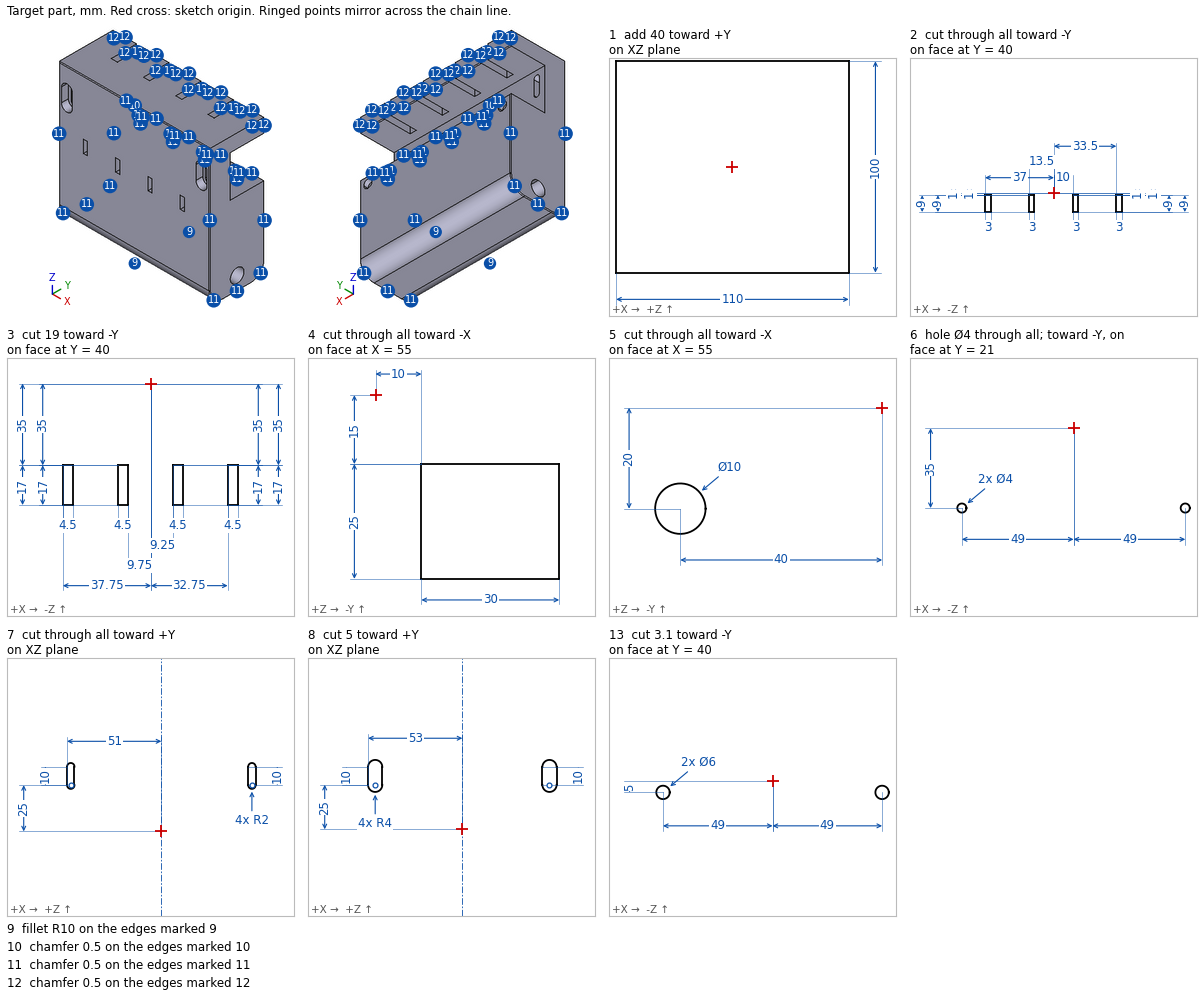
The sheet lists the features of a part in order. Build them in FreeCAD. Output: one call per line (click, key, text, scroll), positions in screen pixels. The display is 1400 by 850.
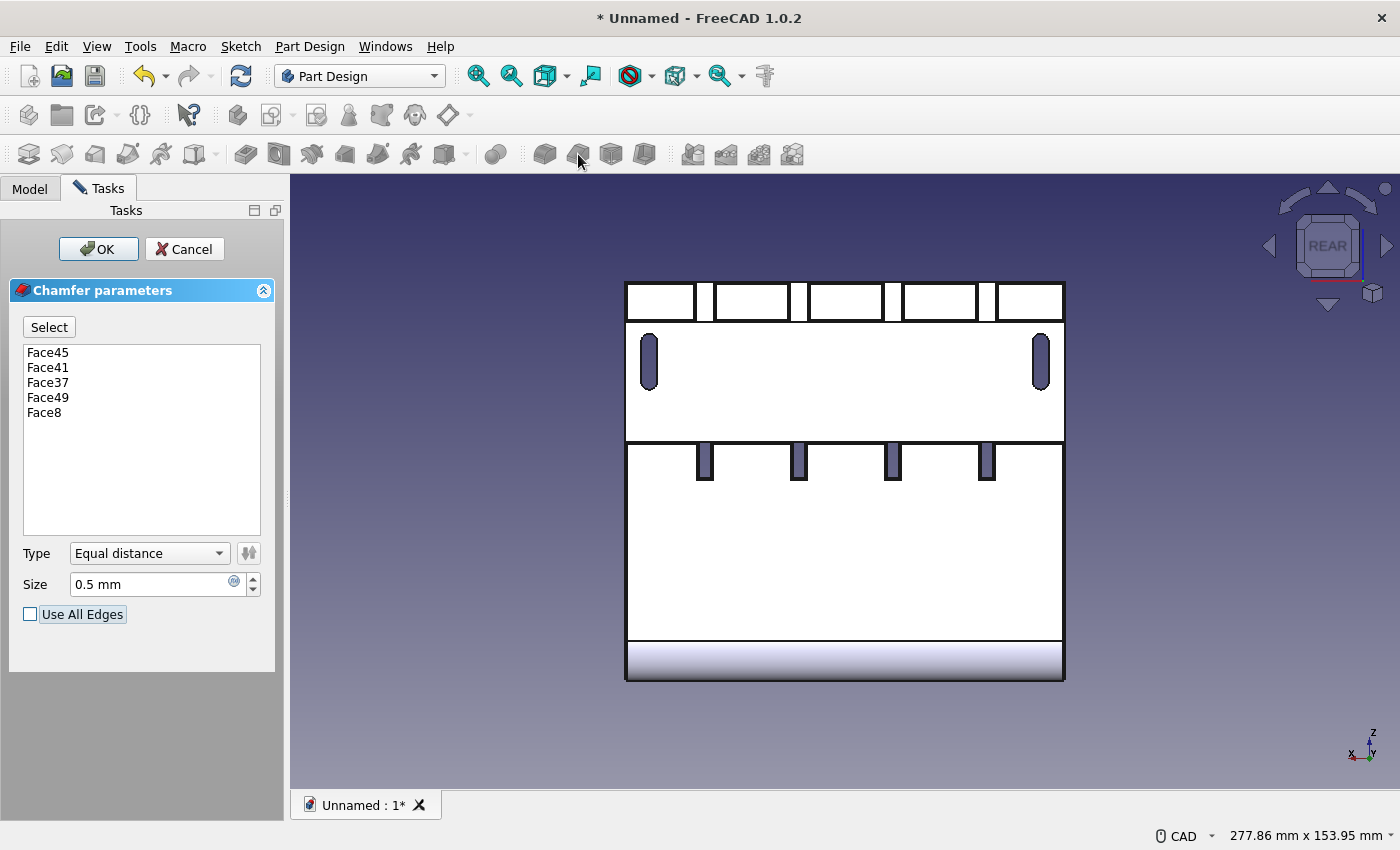
click(99, 249)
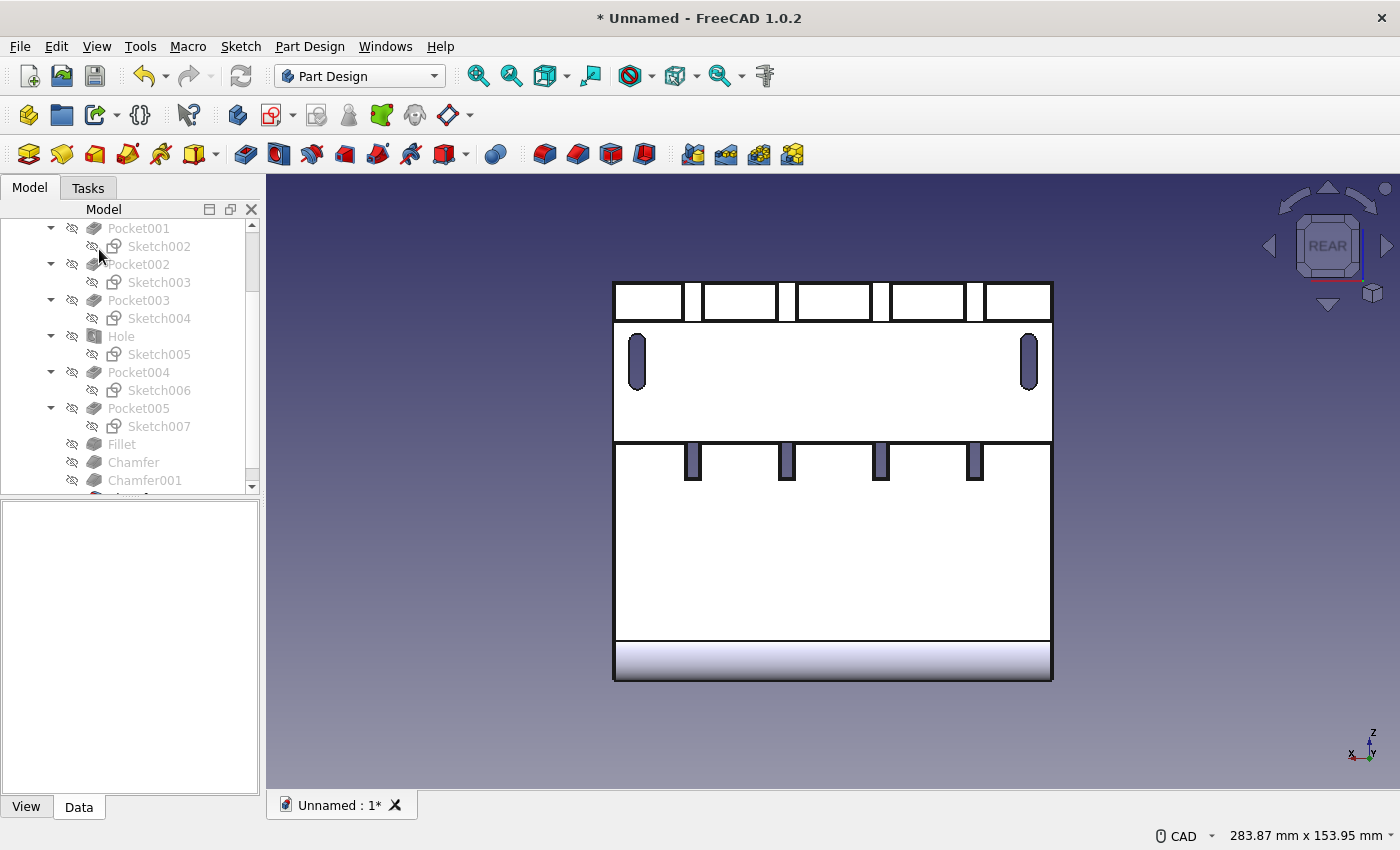
click(833, 541)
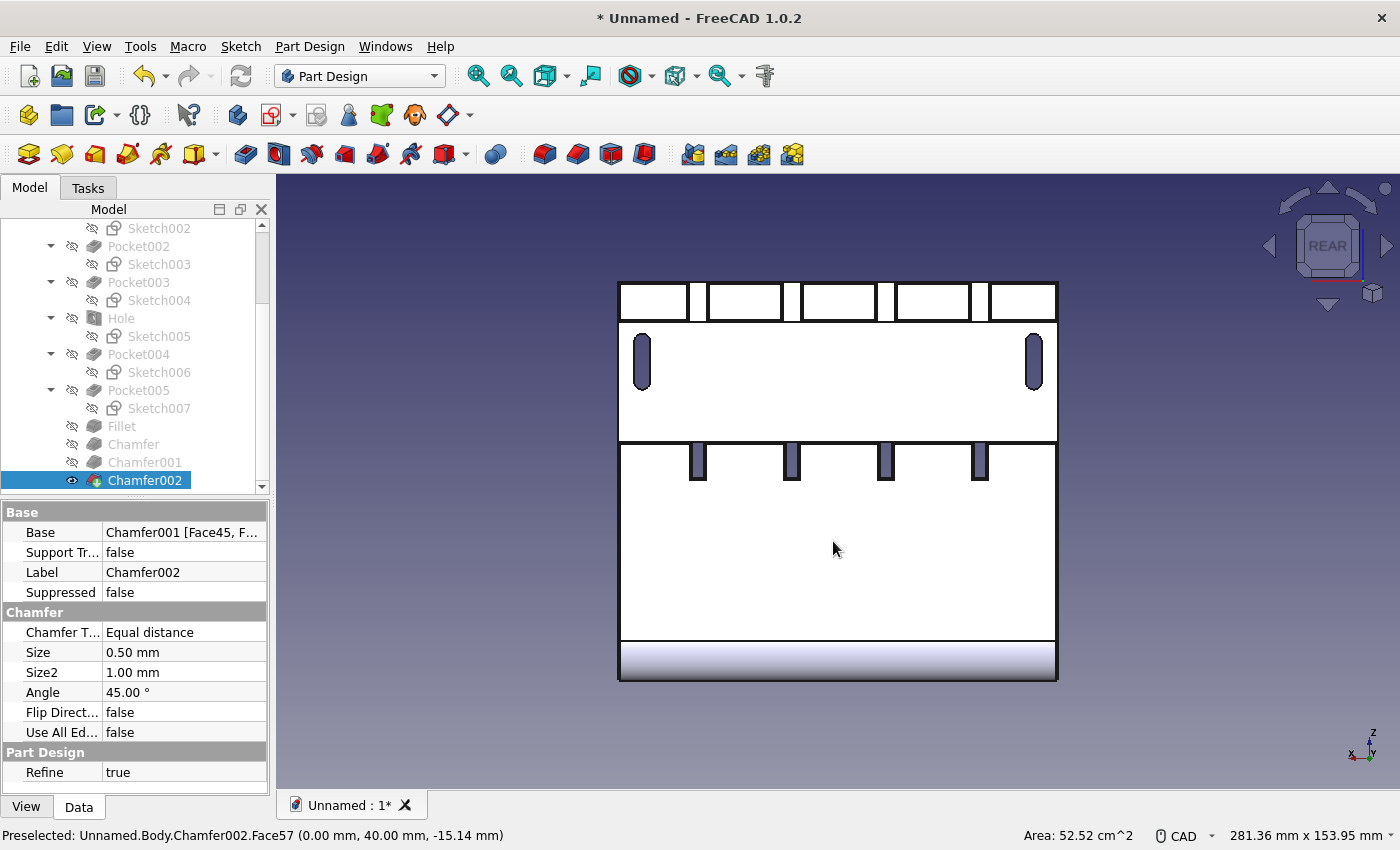
click(270, 116)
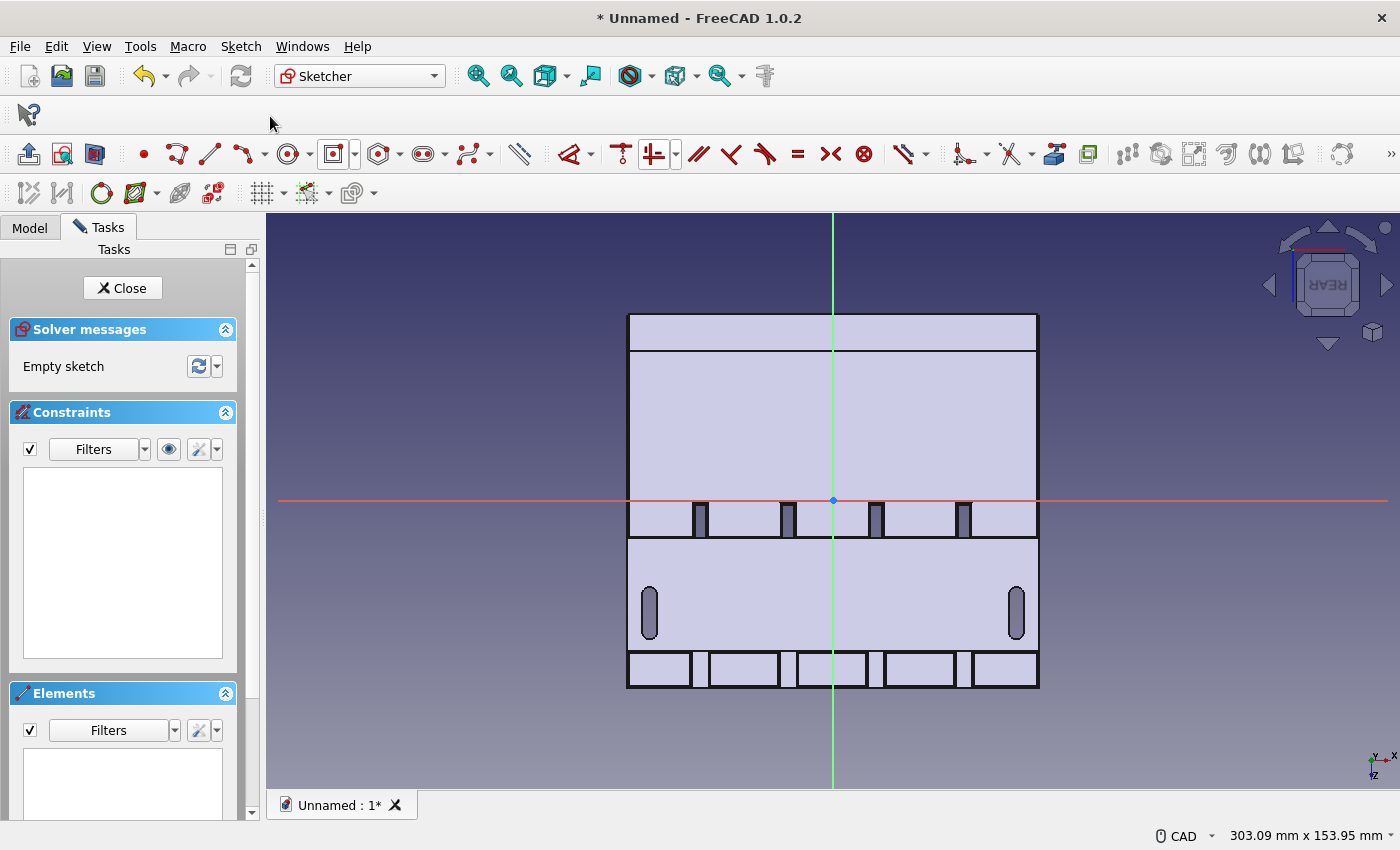
scroll(916, 534, up, 3)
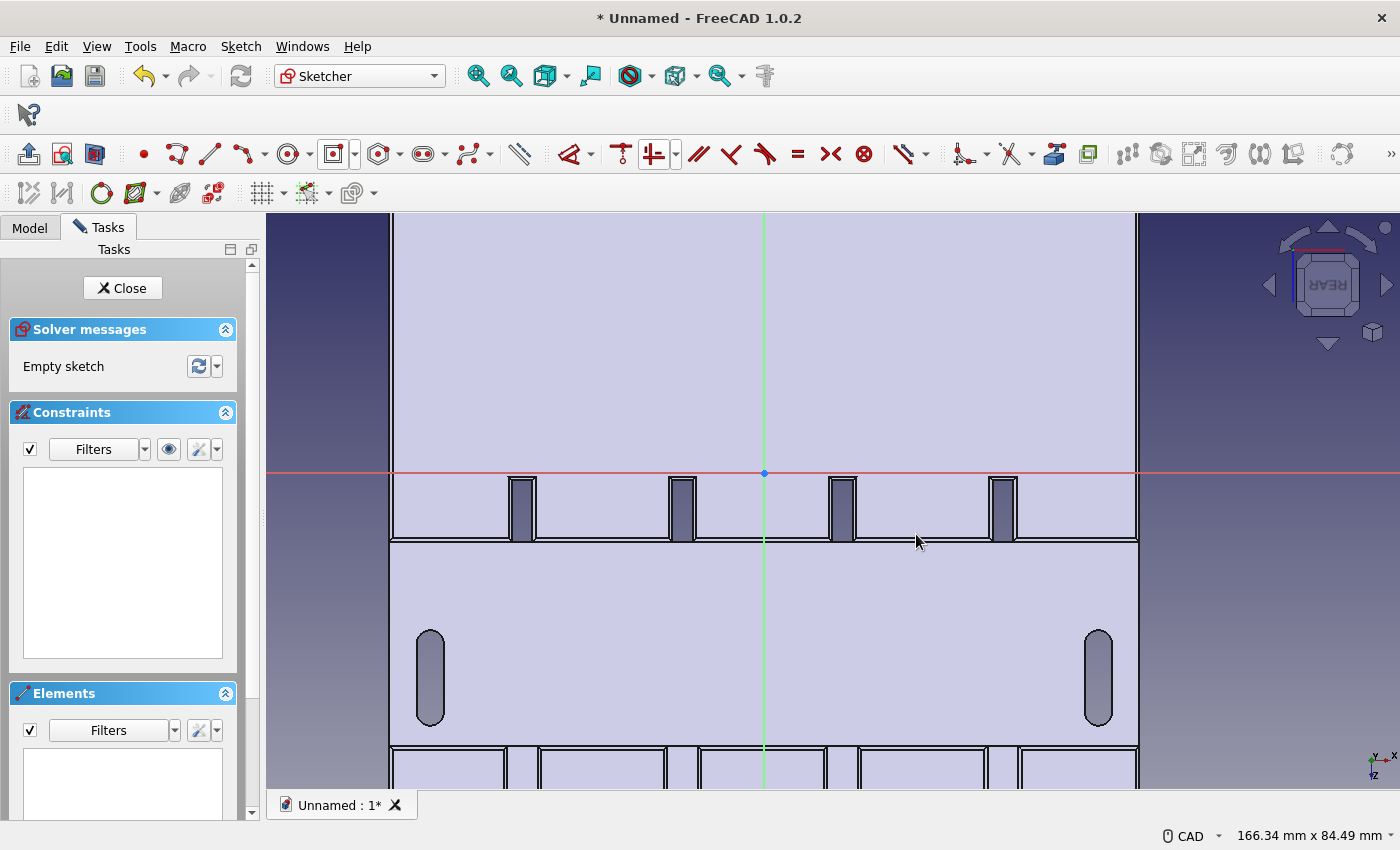
key(g)
key(c)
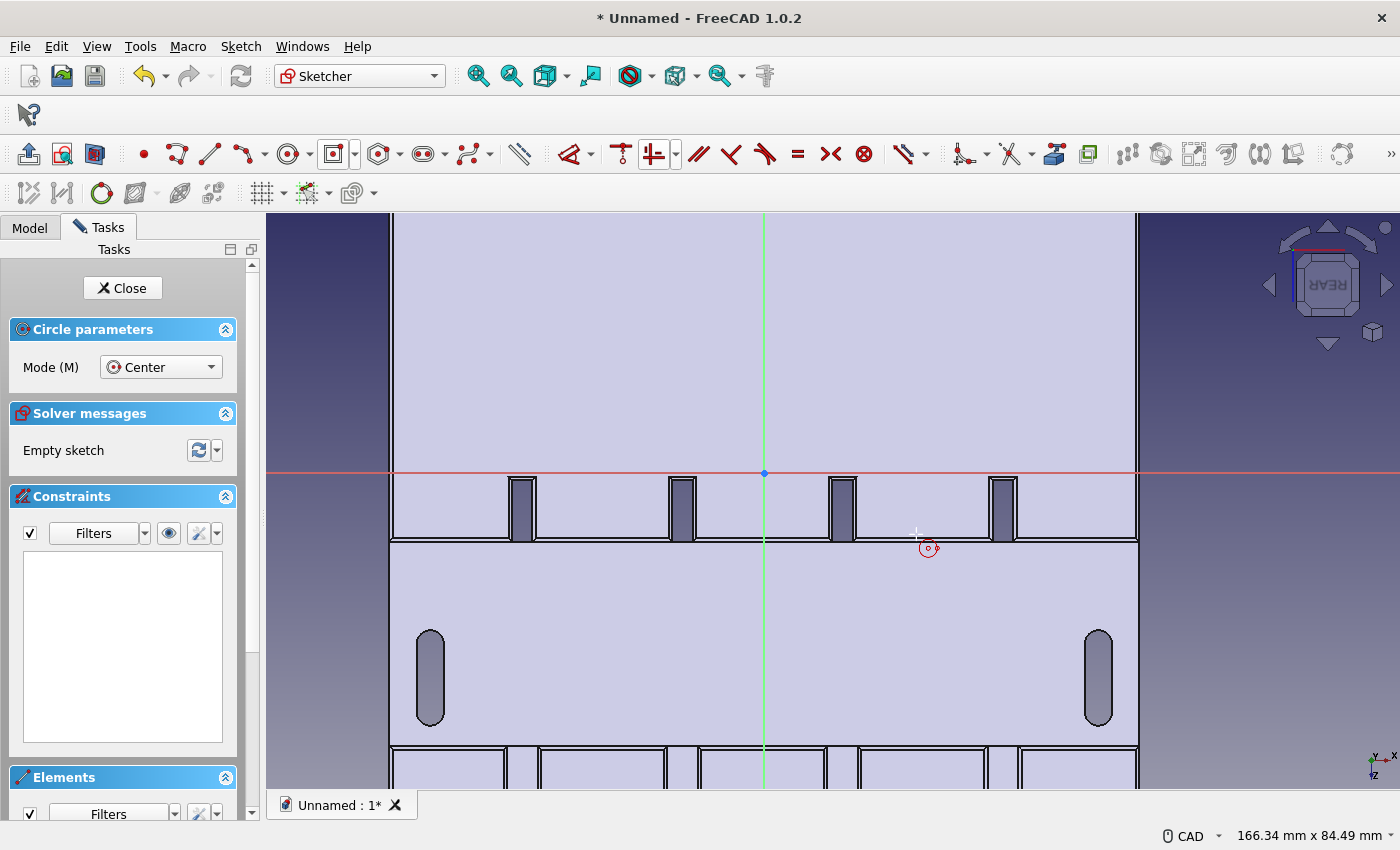
click(430, 507)
click(445, 493)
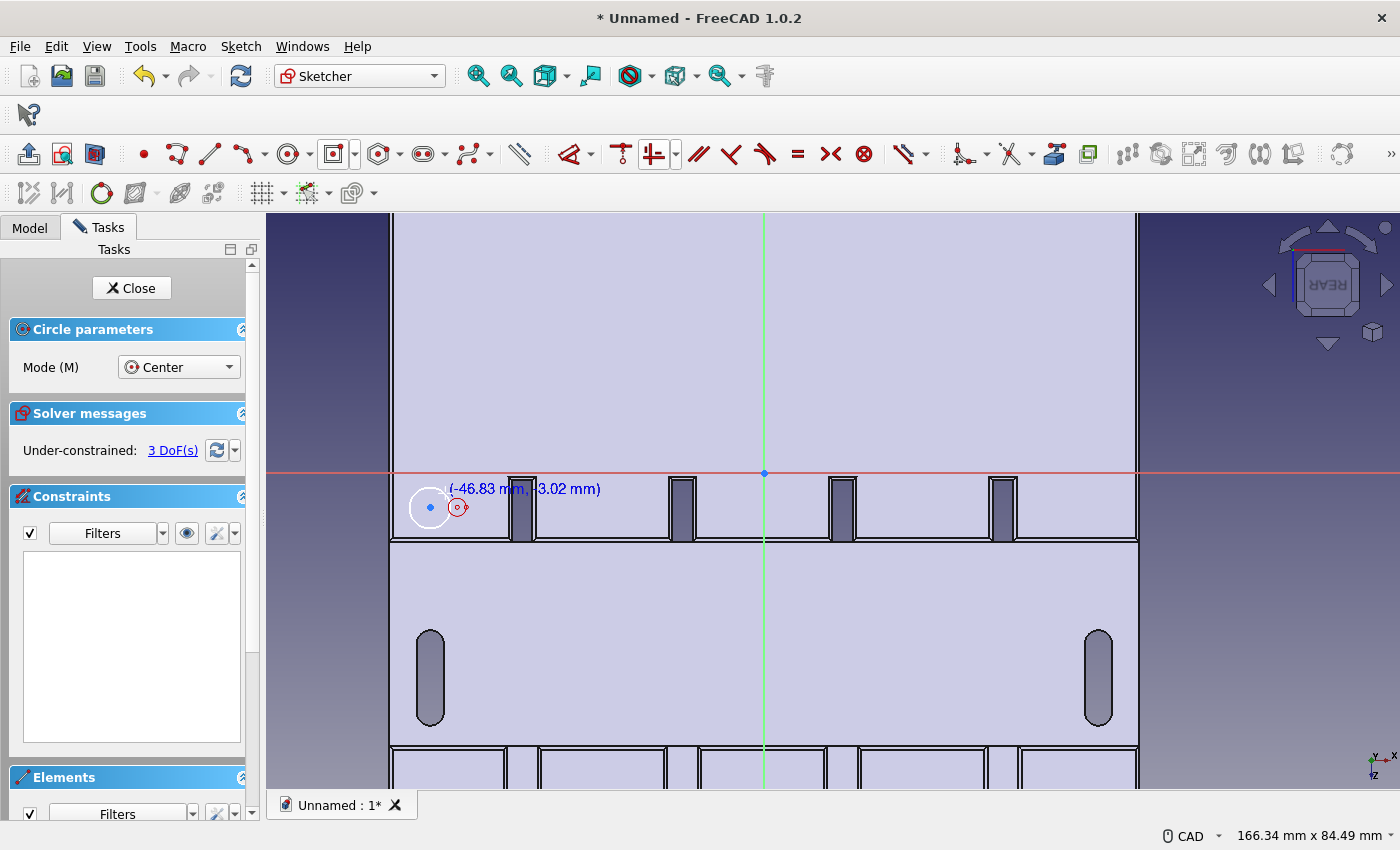
click(1098, 507)
click(1113, 493)
key(Escape)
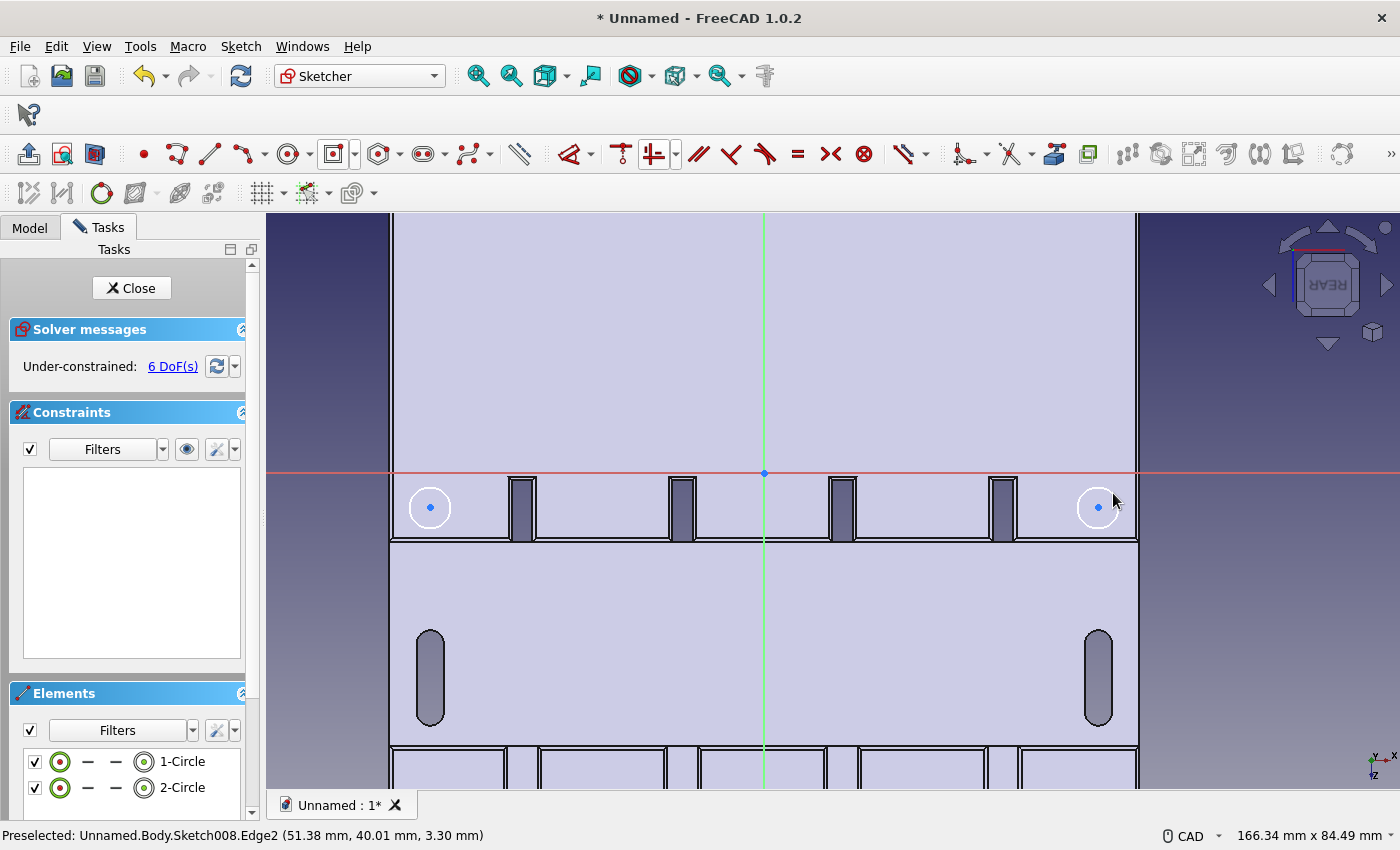
click(444, 493)